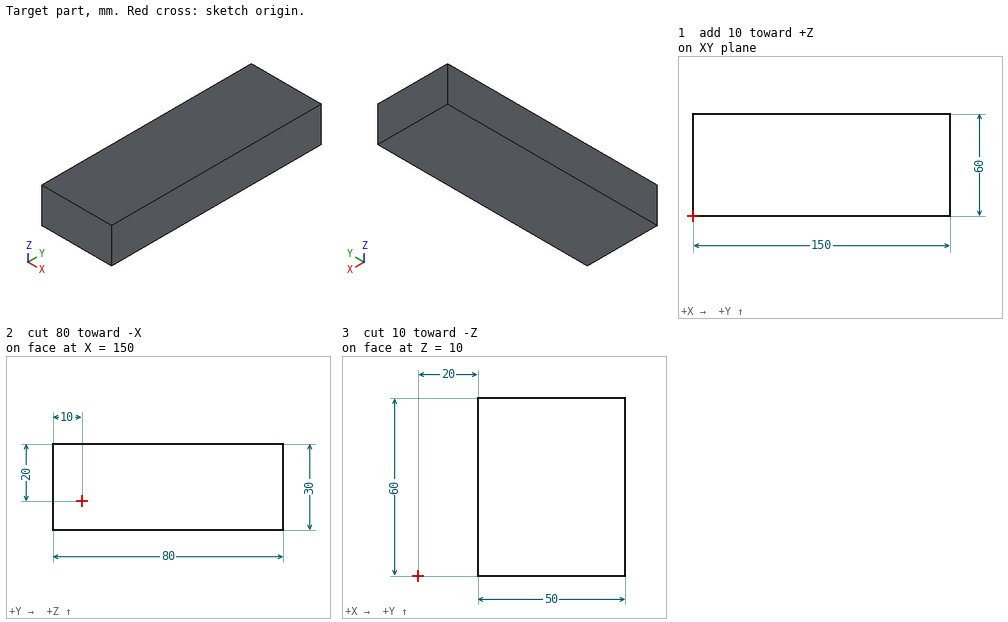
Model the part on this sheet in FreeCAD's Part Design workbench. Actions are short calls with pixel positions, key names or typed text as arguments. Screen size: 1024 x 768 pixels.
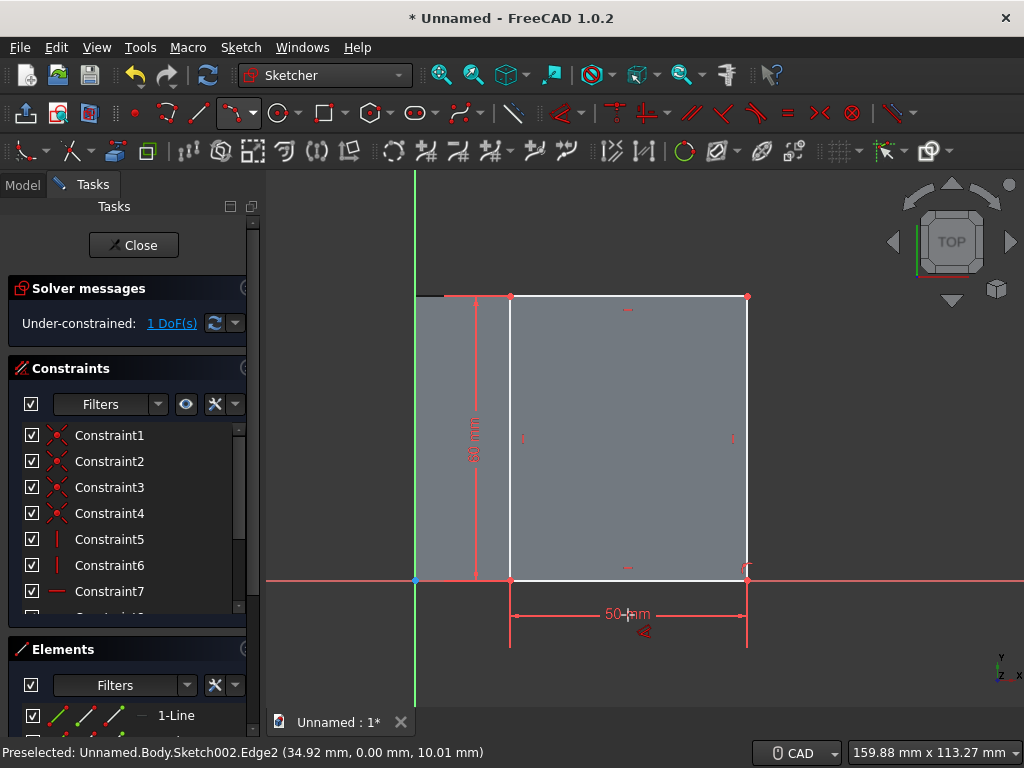
click(510, 296)
click(463, 615)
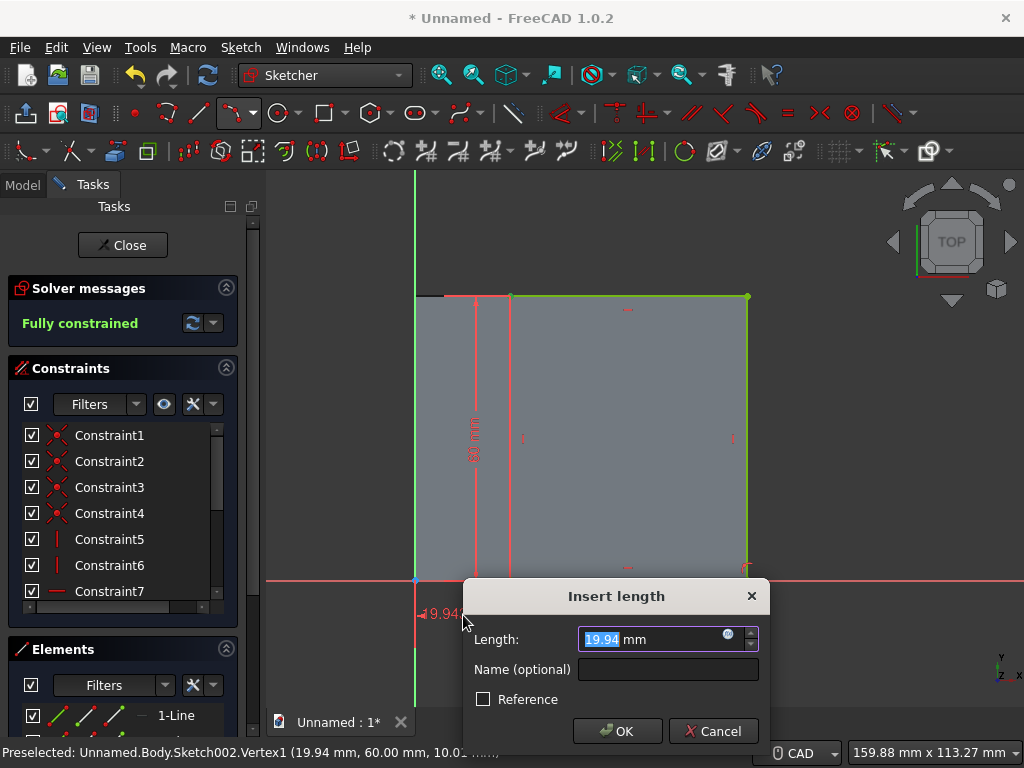
text(20)
key(Return)
key(Escape)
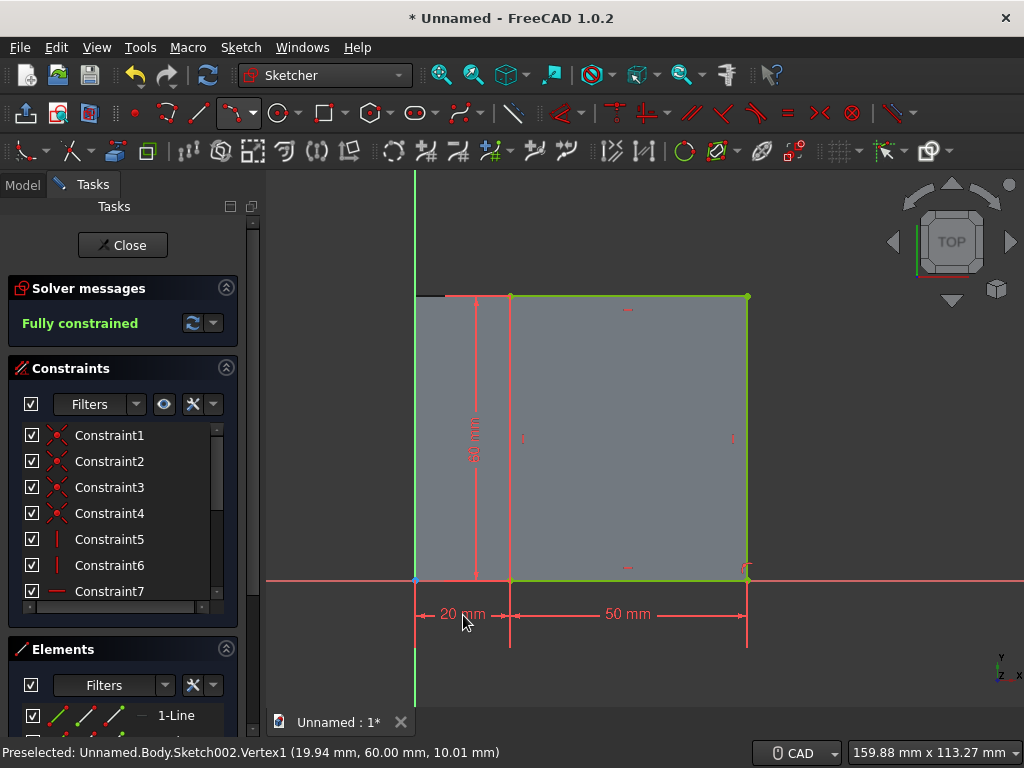
click(123, 245)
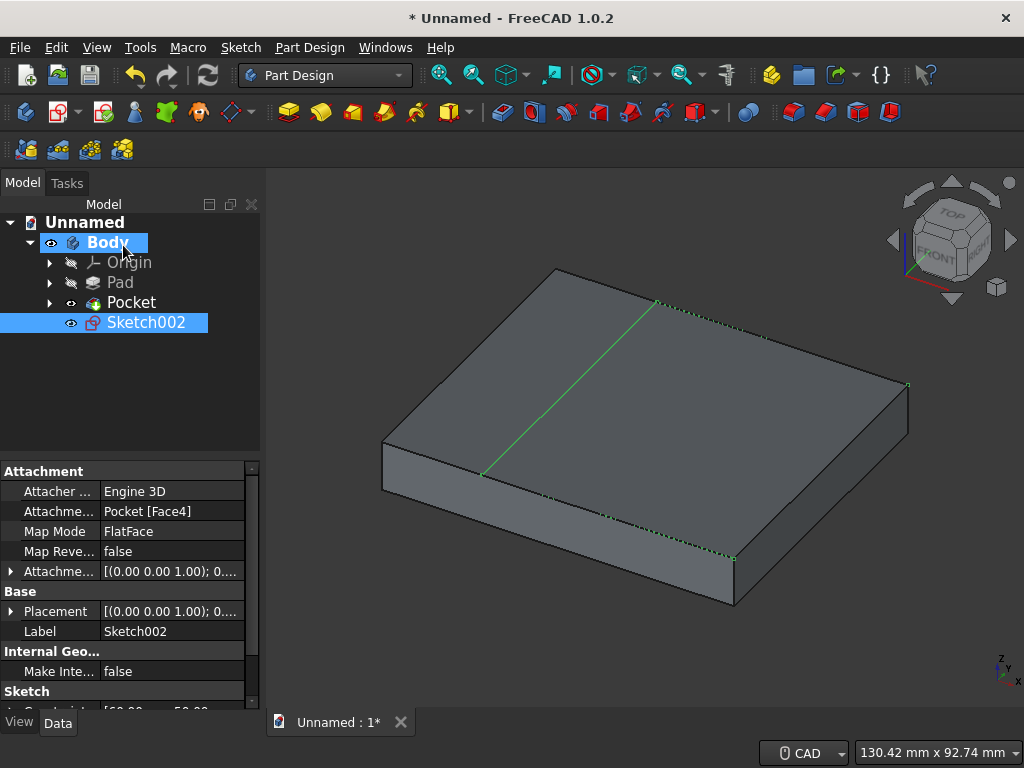
click(504, 112)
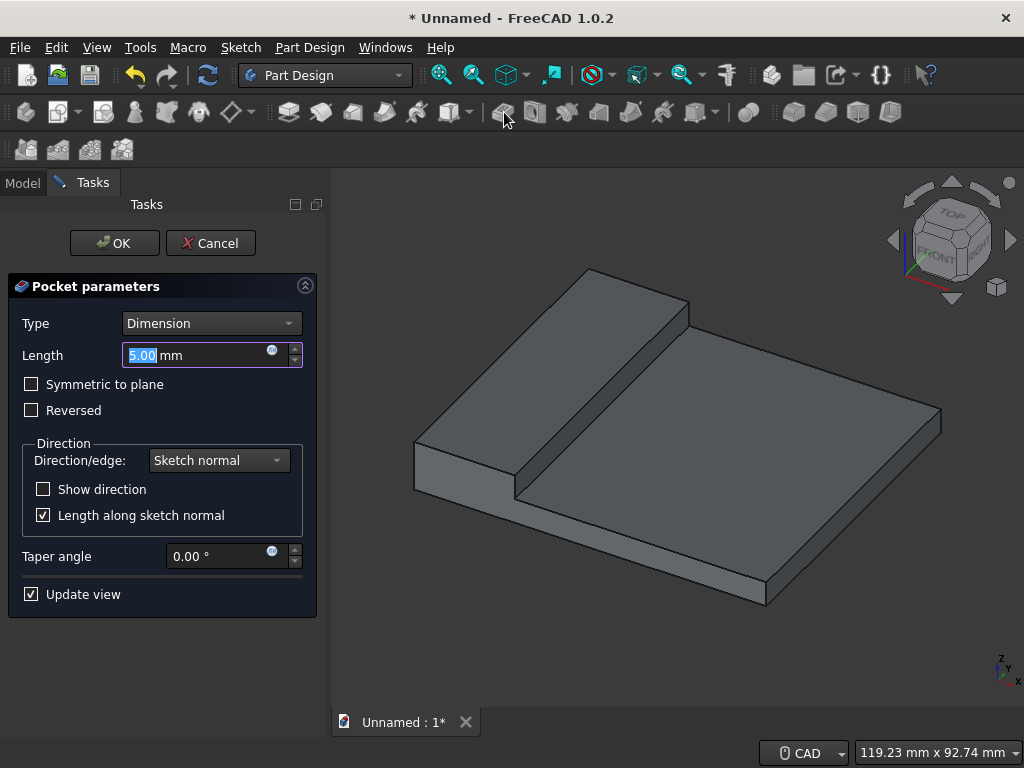
text(10)
key(Tab)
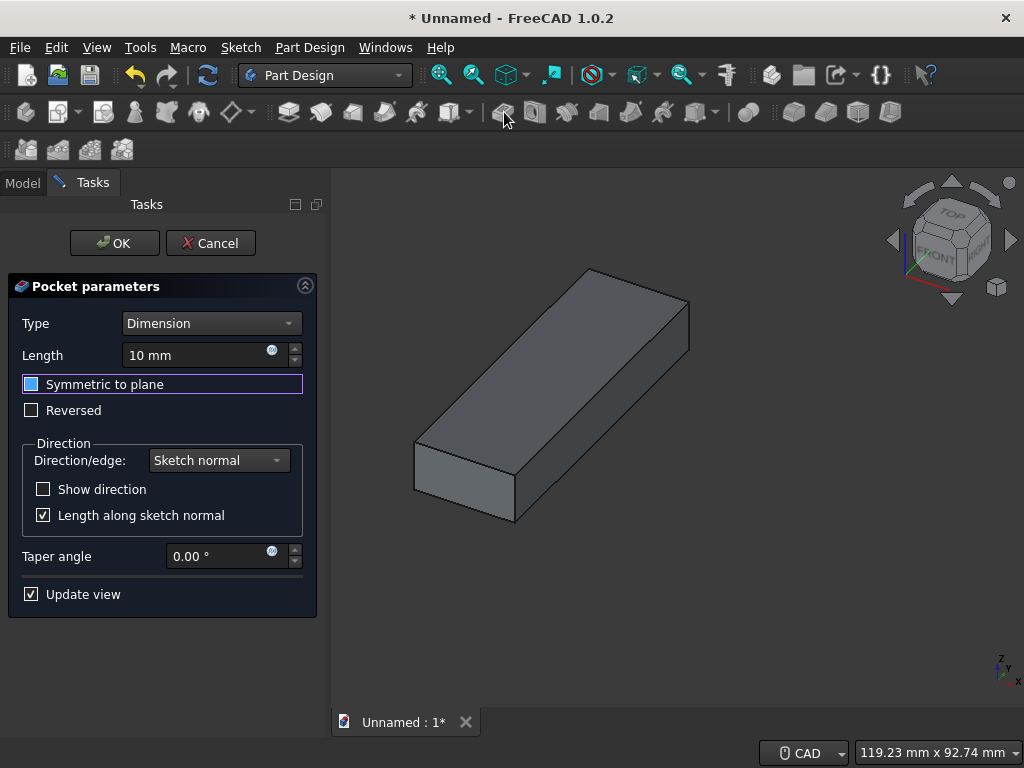
click(115, 243)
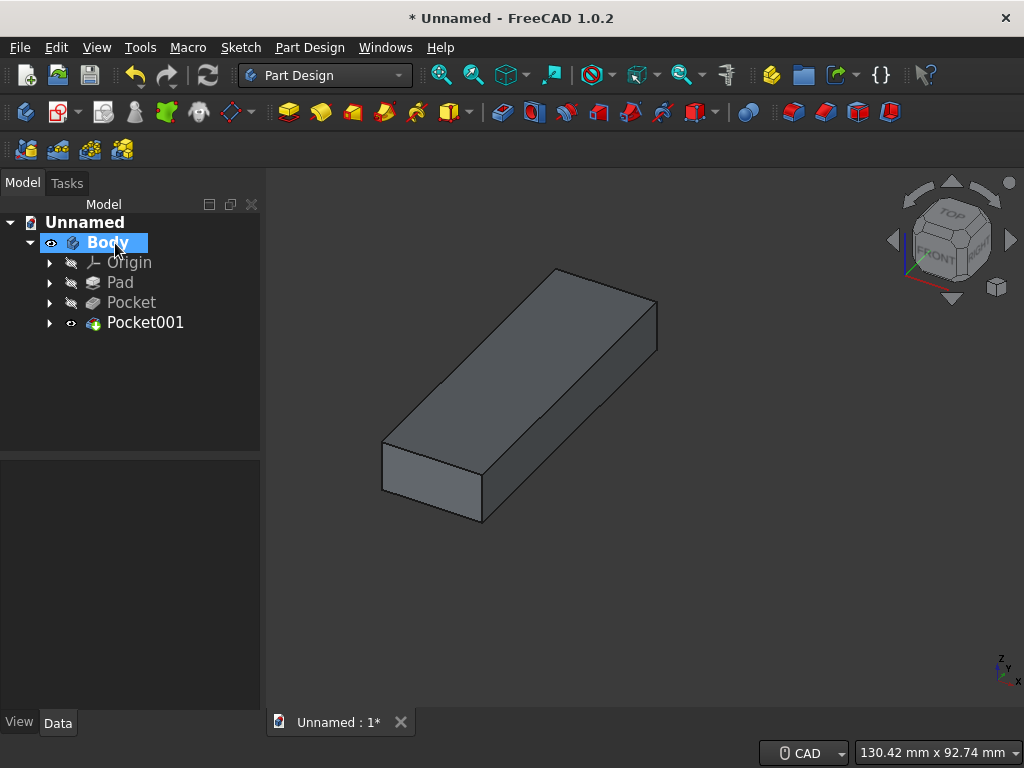
key(0)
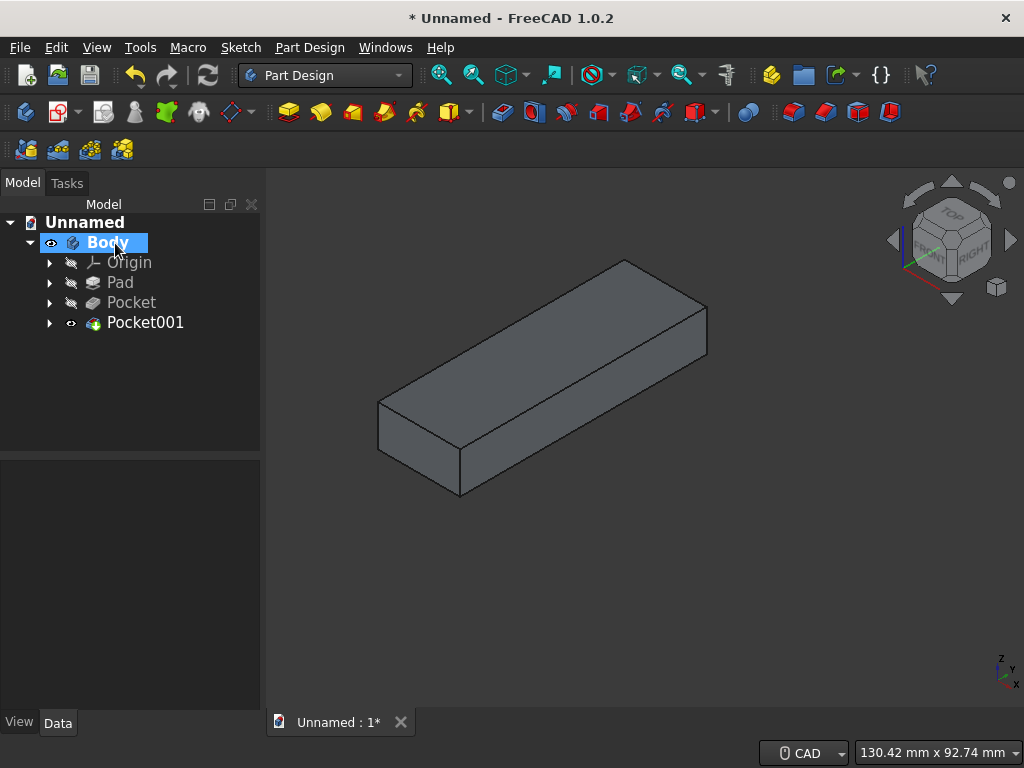
click(442, 76)